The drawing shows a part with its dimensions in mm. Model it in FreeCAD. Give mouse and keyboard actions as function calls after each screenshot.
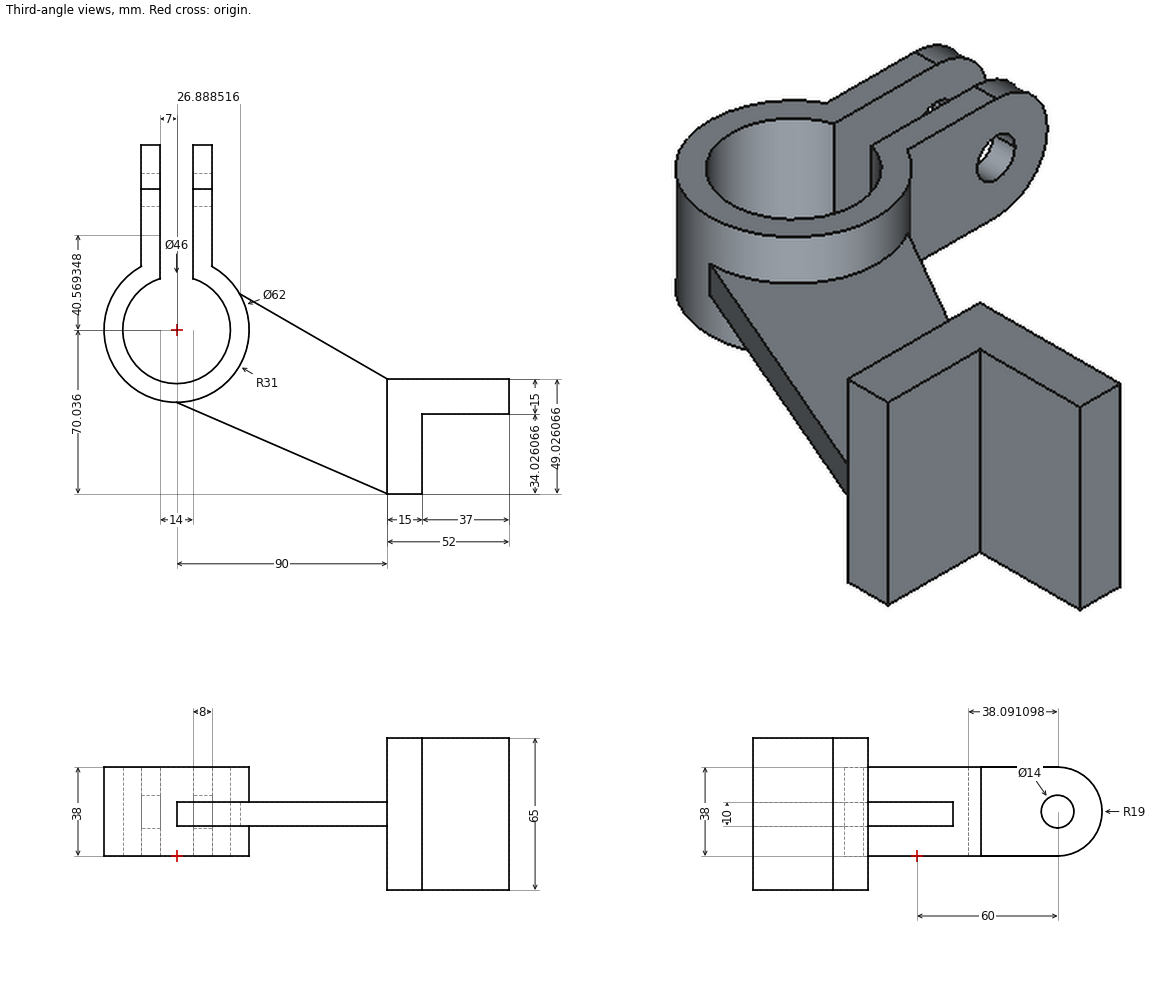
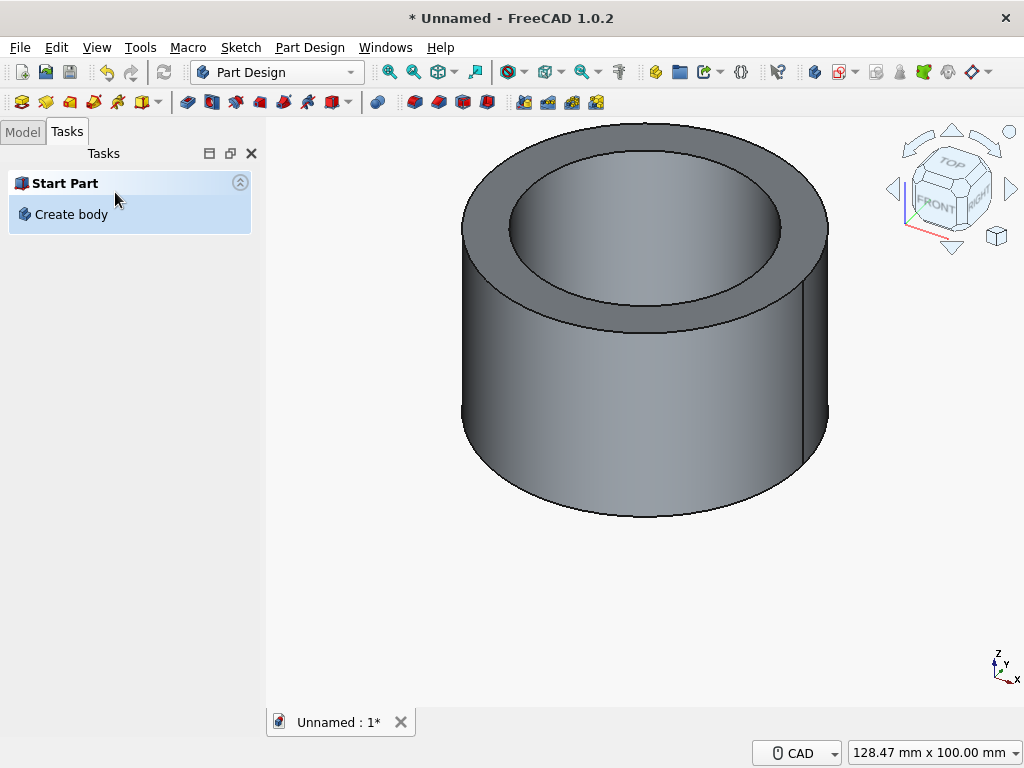
click(390, 72)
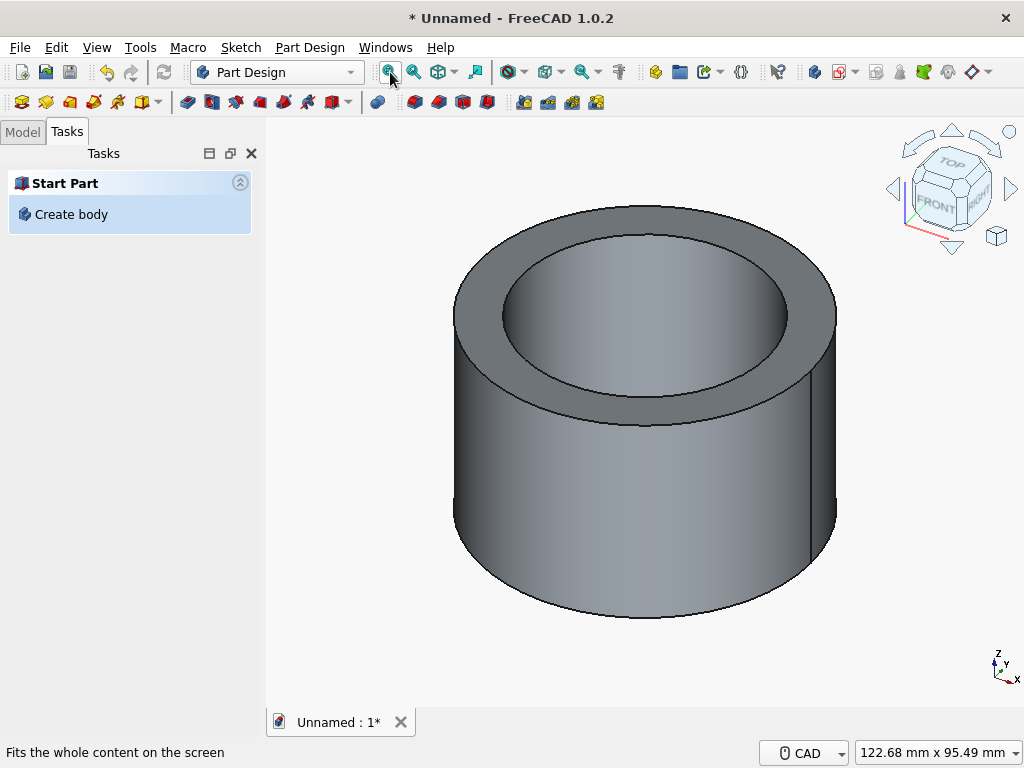
click(787, 362)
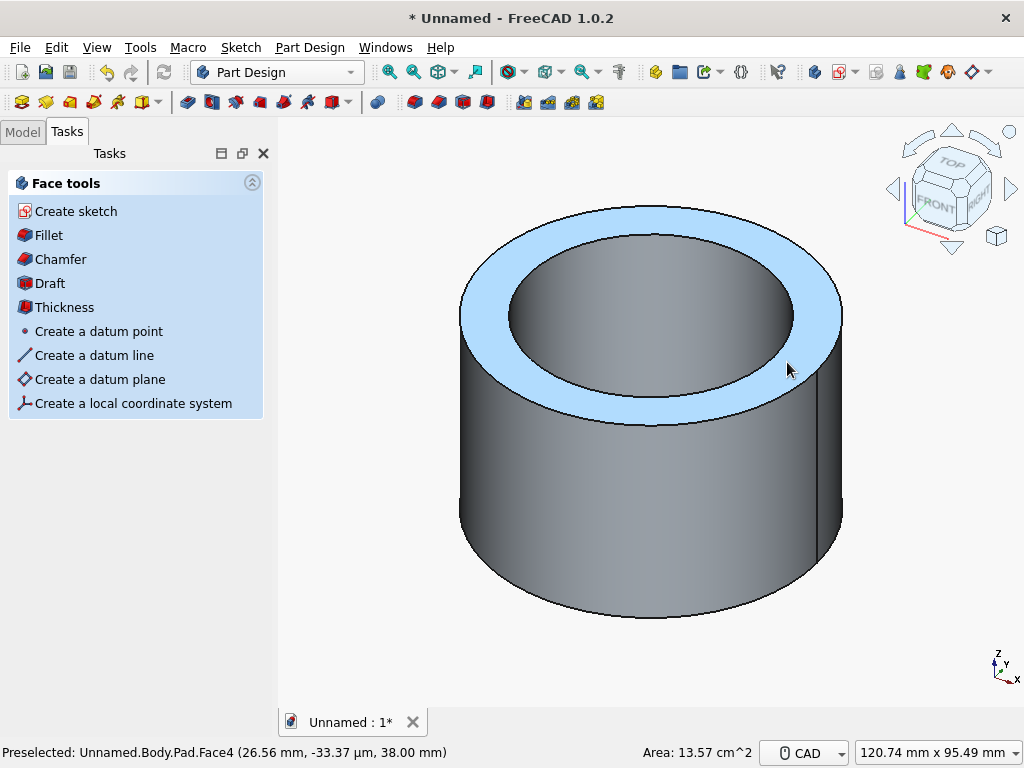
click(840, 72)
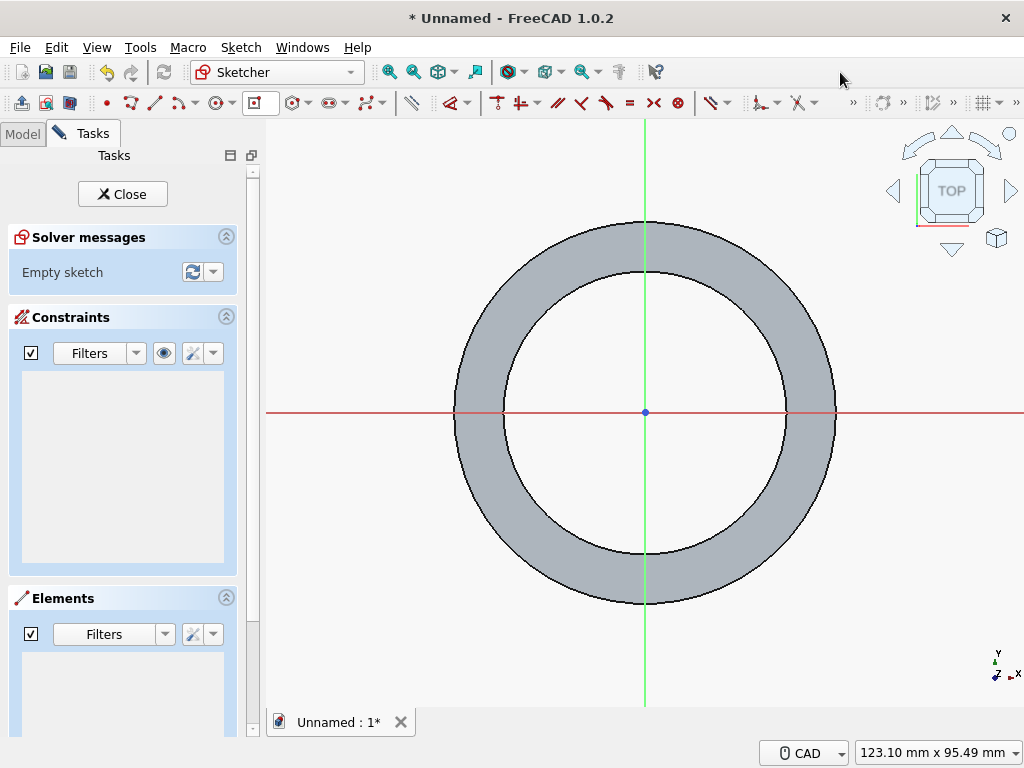
scroll(294, 679, down, 1)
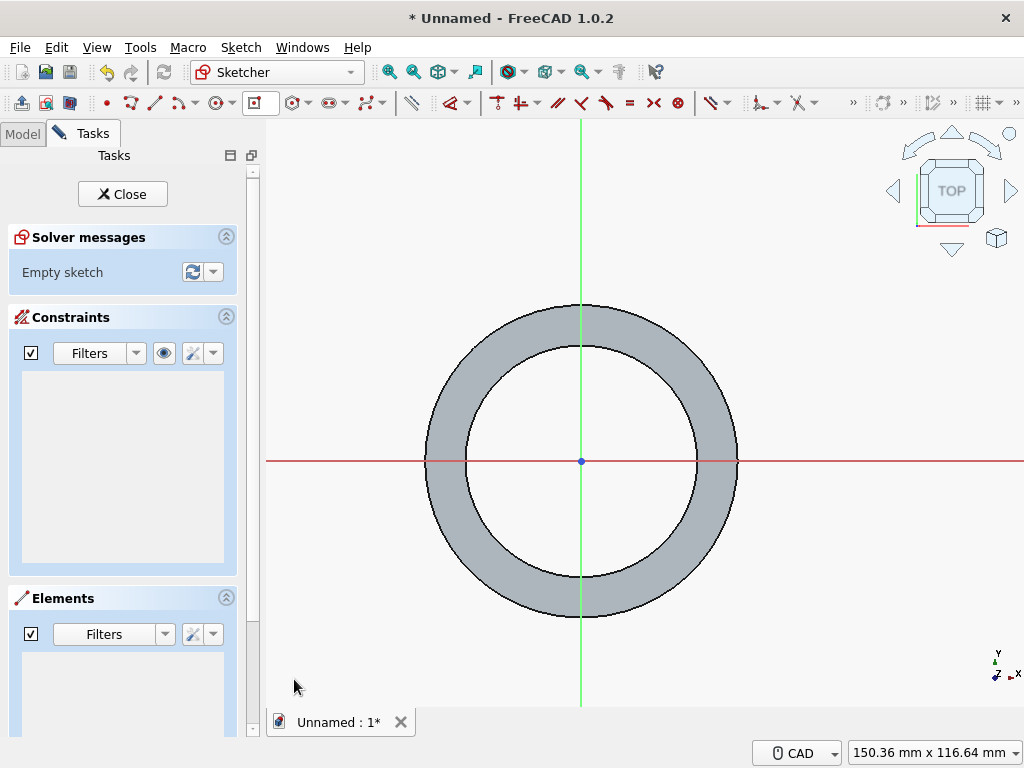
scroll(587, 294, up, 3)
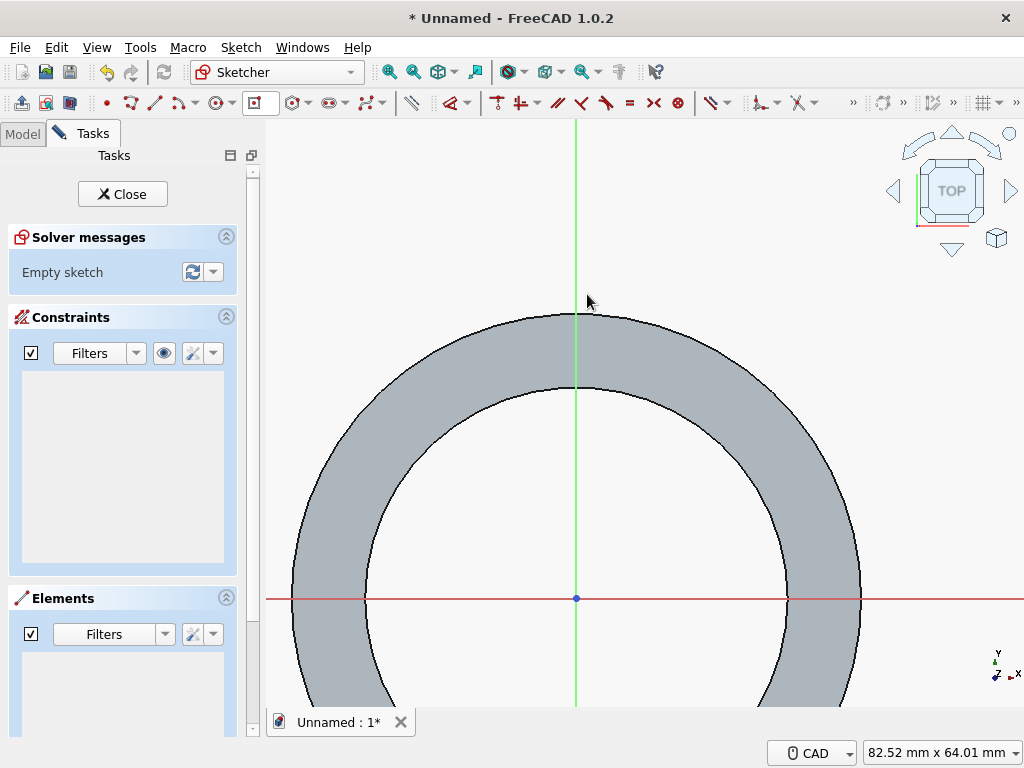
key(g)
key(r)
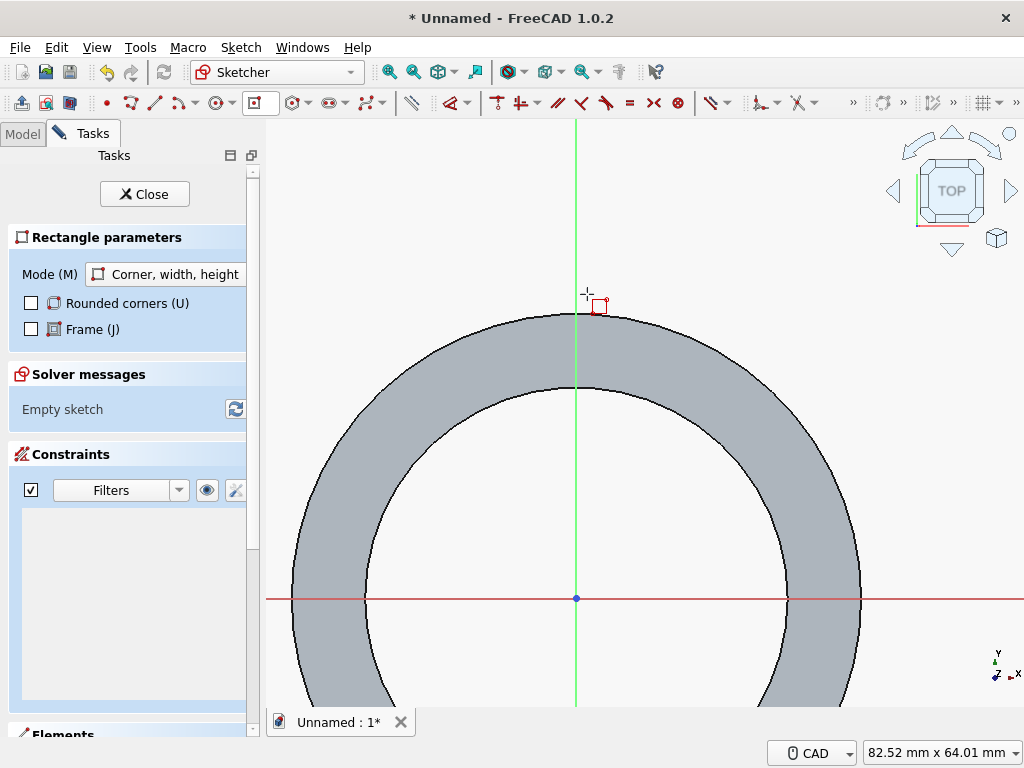
click(512, 226)
click(641, 599)
key(Escape)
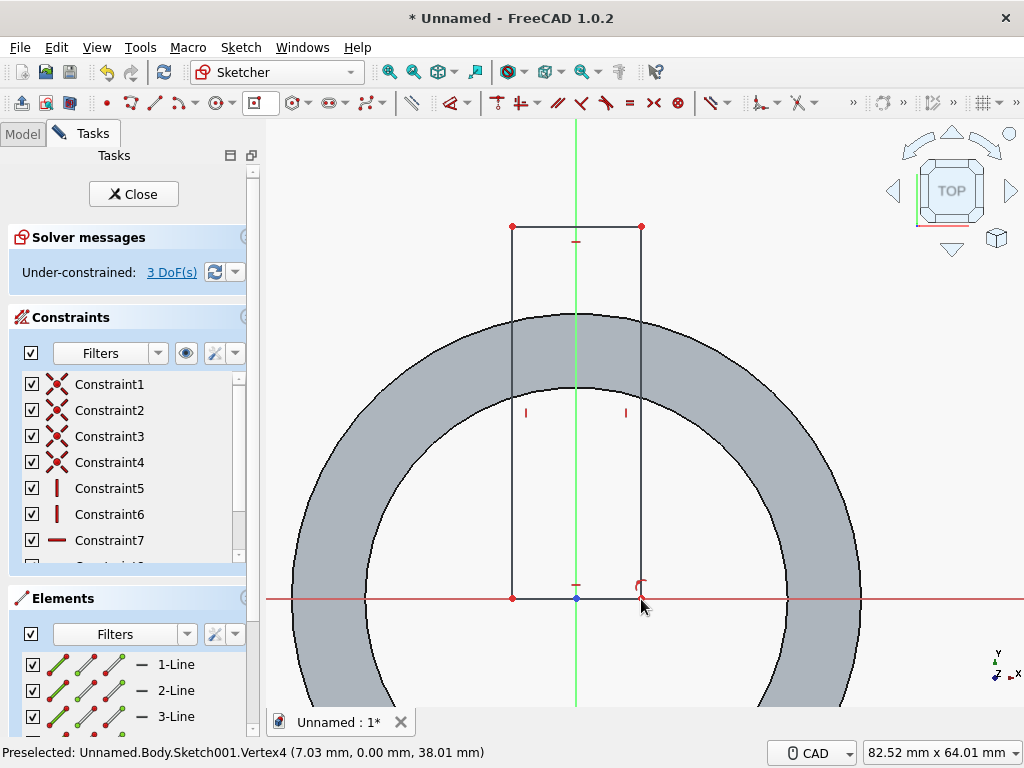
key(d)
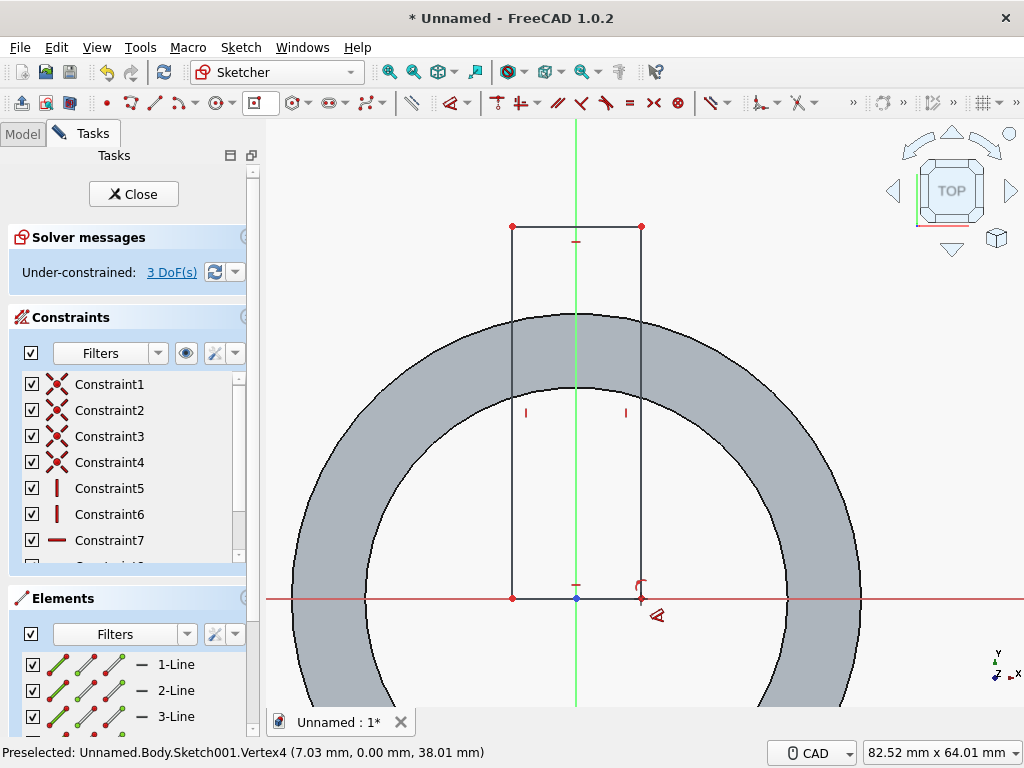
click(551, 599)
click(547, 633)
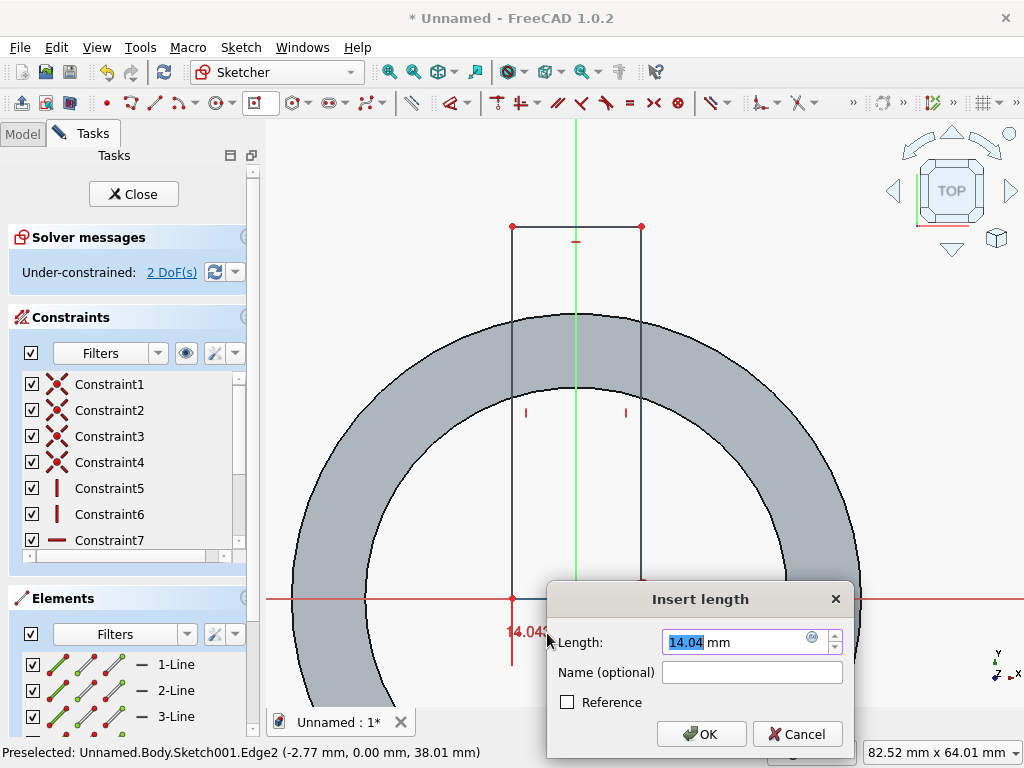
text(14)
key(Return)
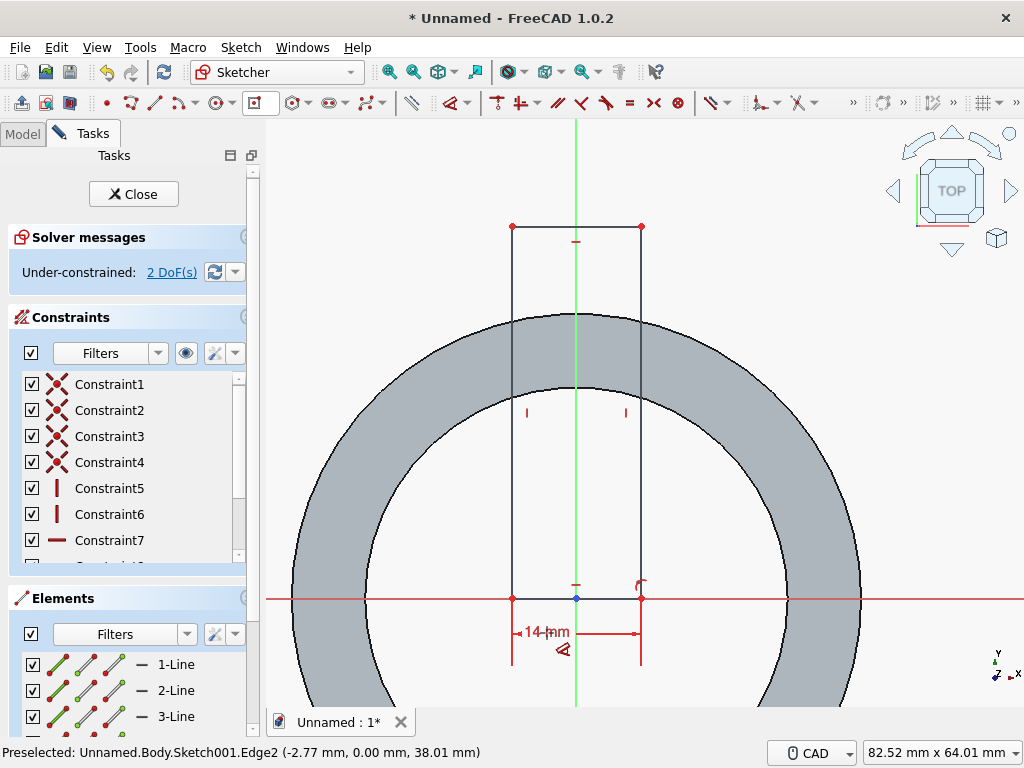
click(512, 227)
click(544, 193)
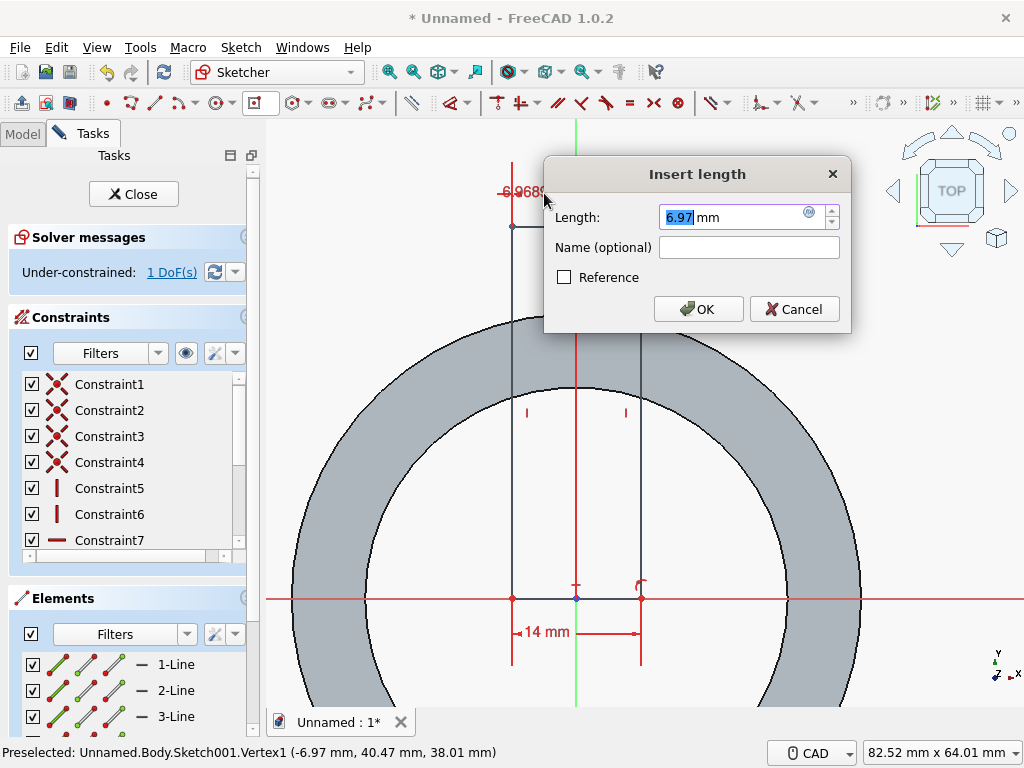
text(7)
key(Return)